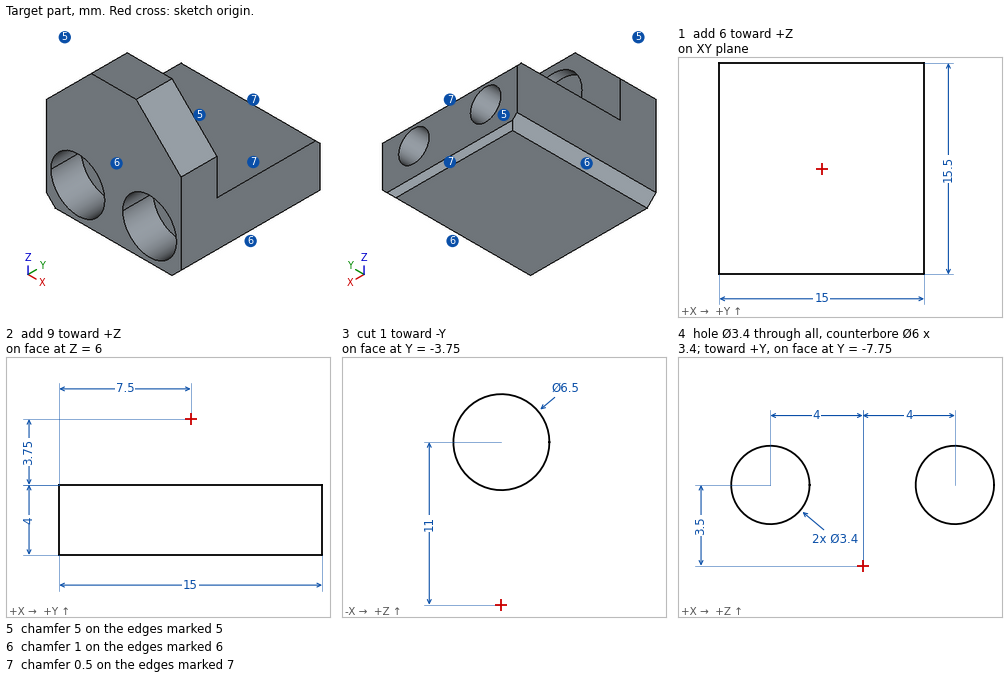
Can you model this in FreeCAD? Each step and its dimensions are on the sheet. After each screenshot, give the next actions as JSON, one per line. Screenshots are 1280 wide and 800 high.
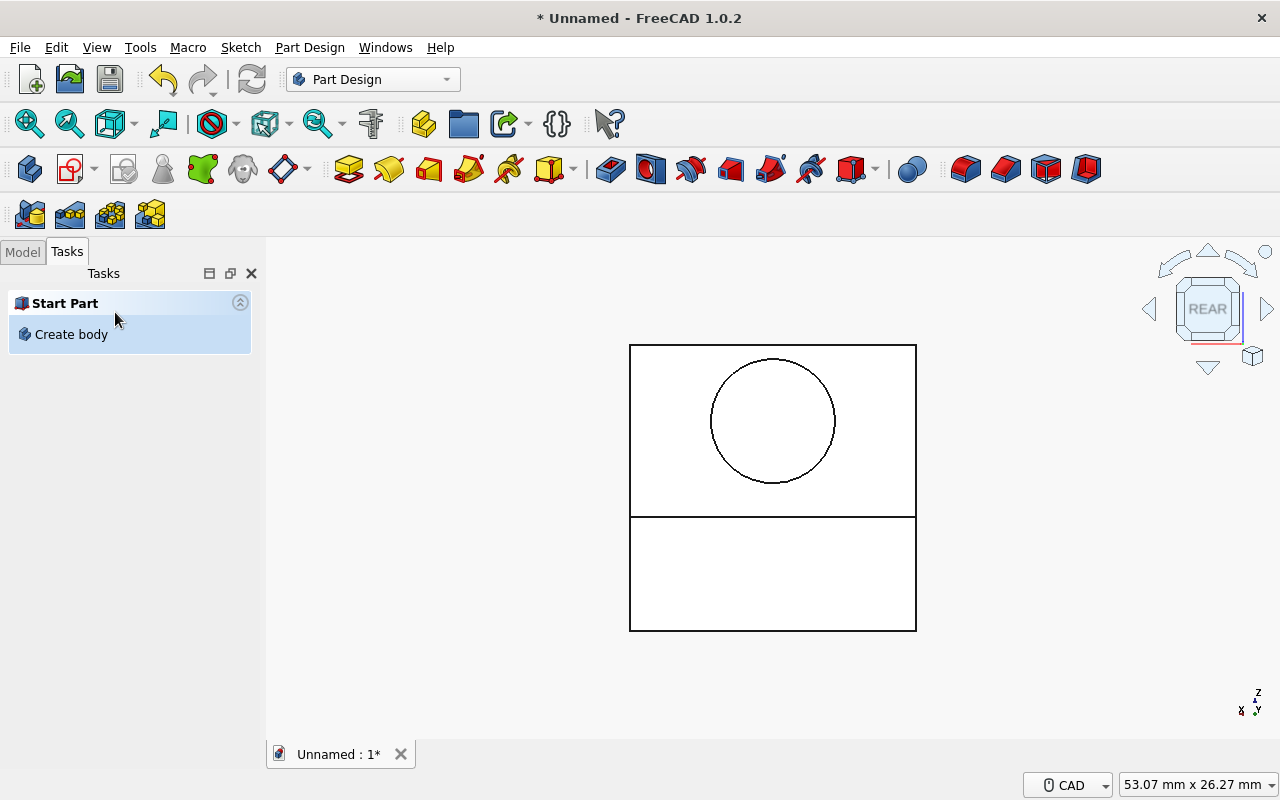
{"action": "key", "text": "0"}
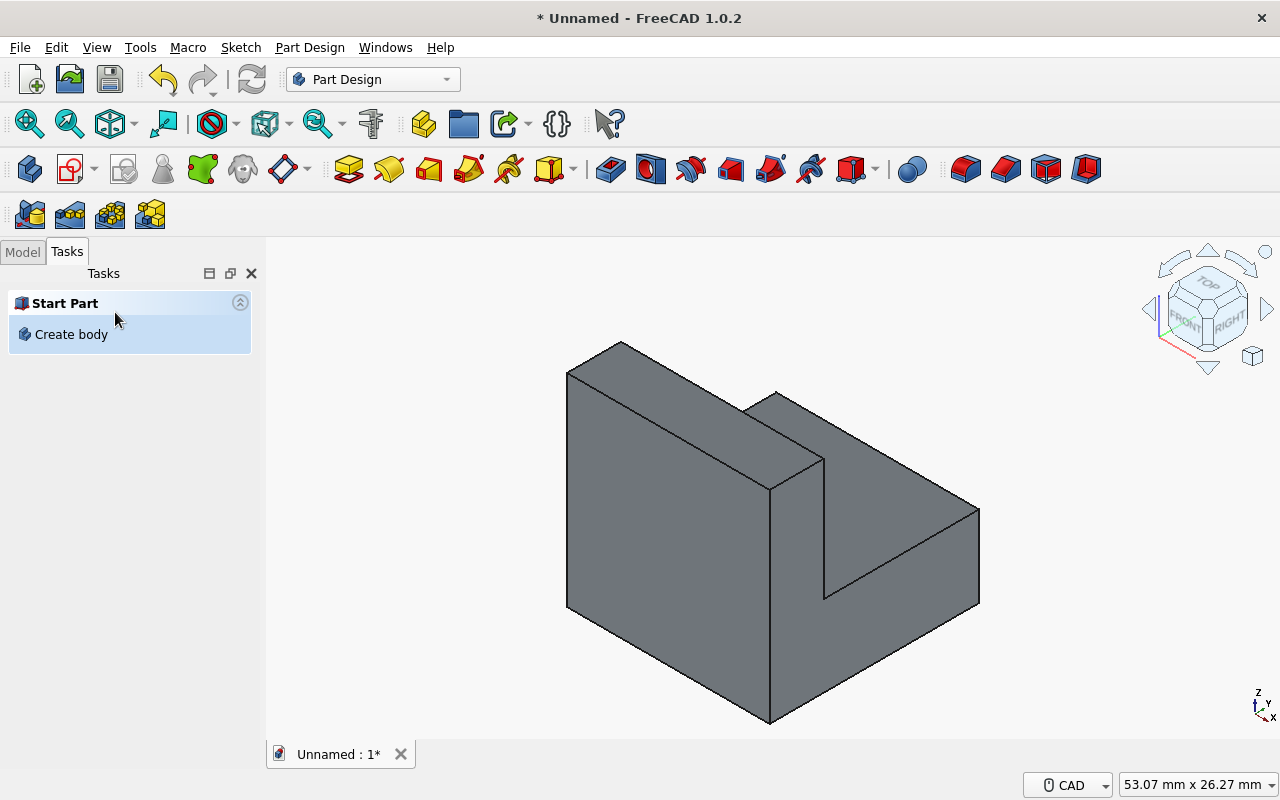
{"action": "left_click", "coordinate": [668, 547]}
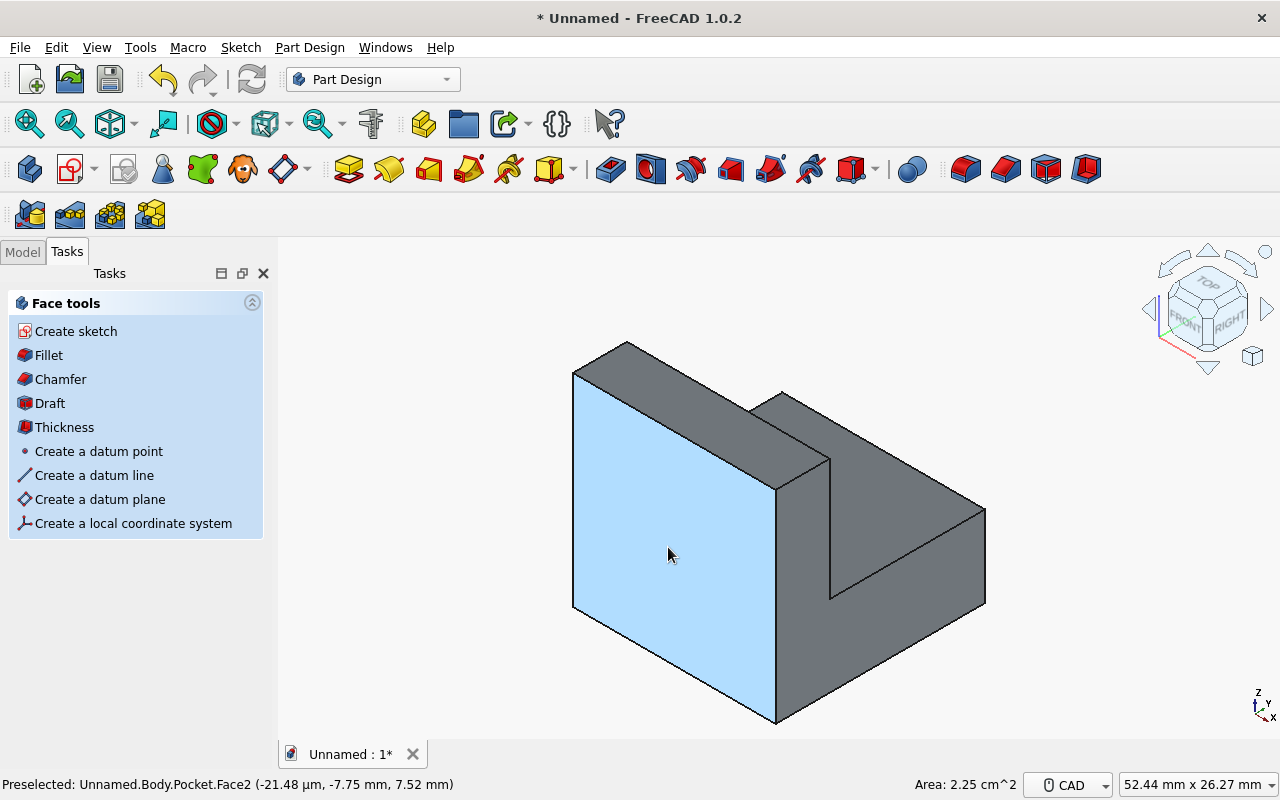
{"action": "left_click", "coordinate": [70, 170]}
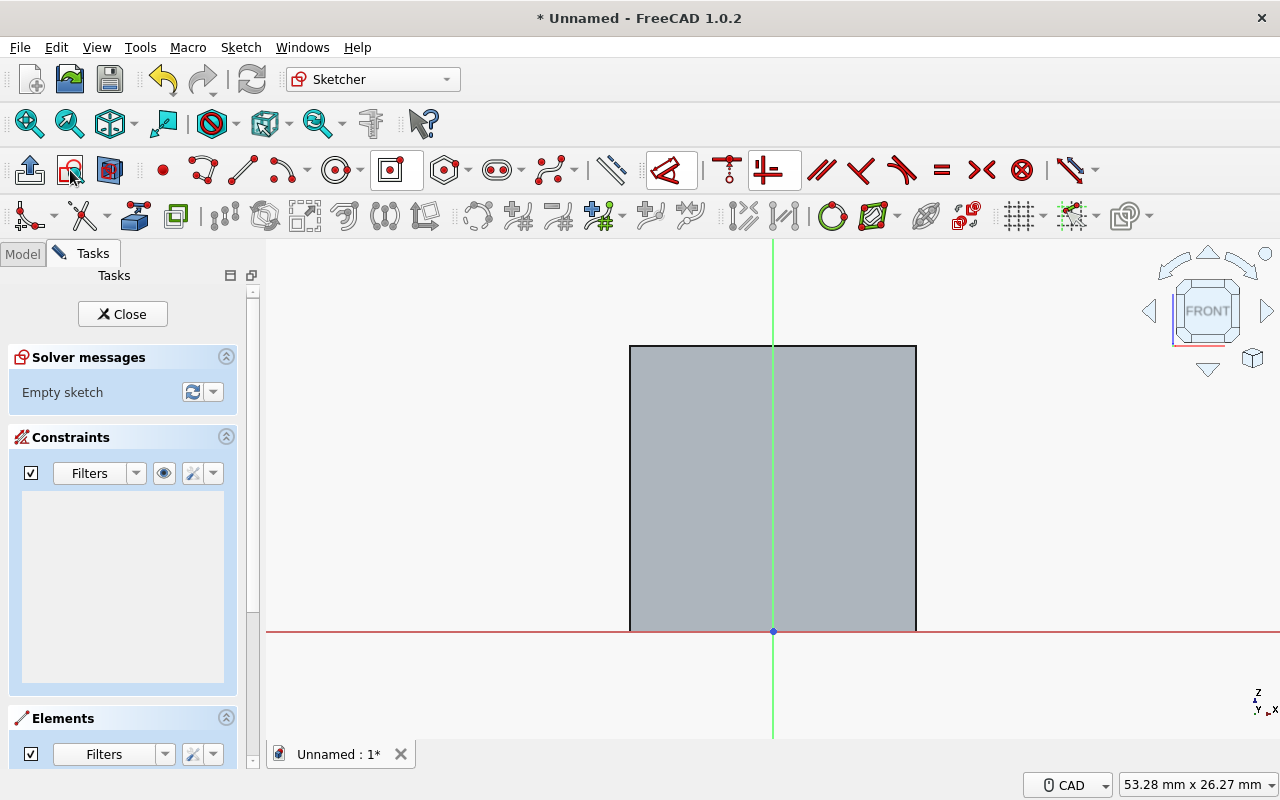
{"action": "scroll", "coordinate": [813, 637], "scroll_direction": "up", "scroll_amount": 5}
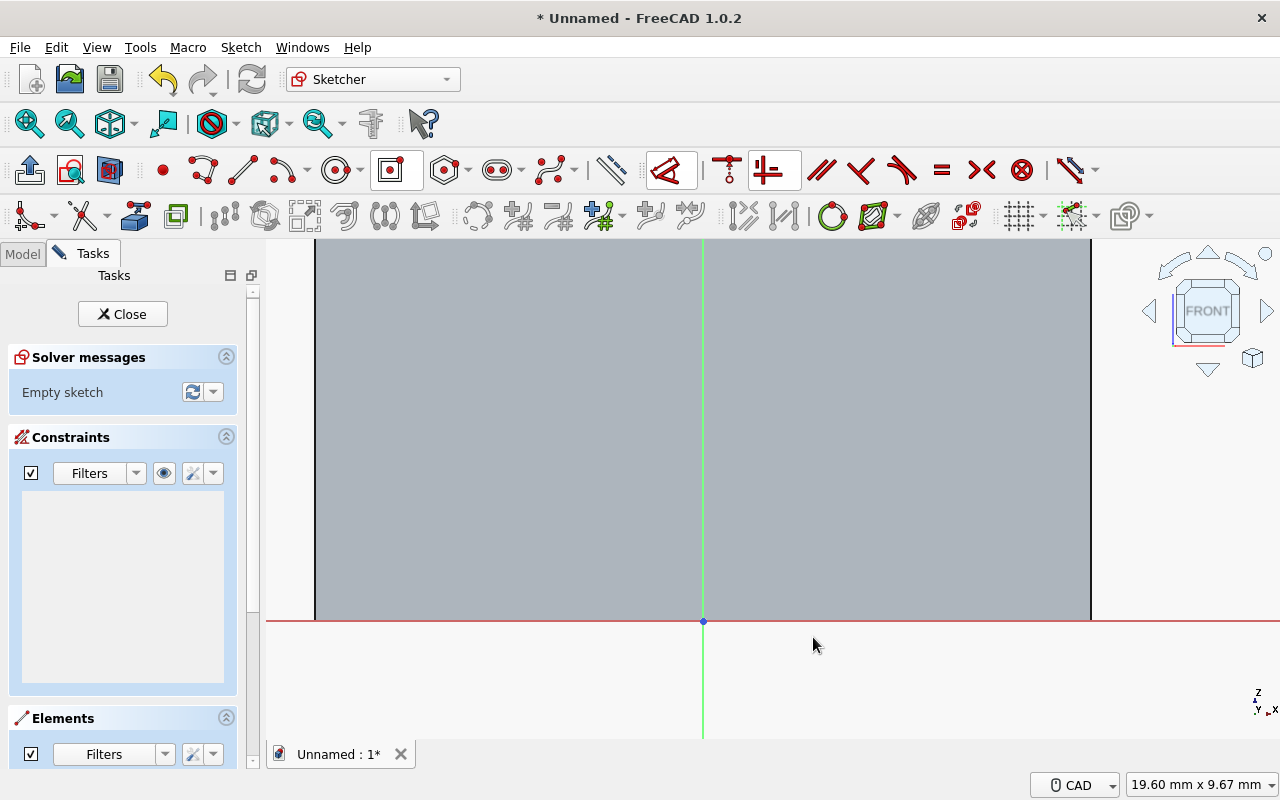
{"action": "left_click", "coordinate": [336, 170]}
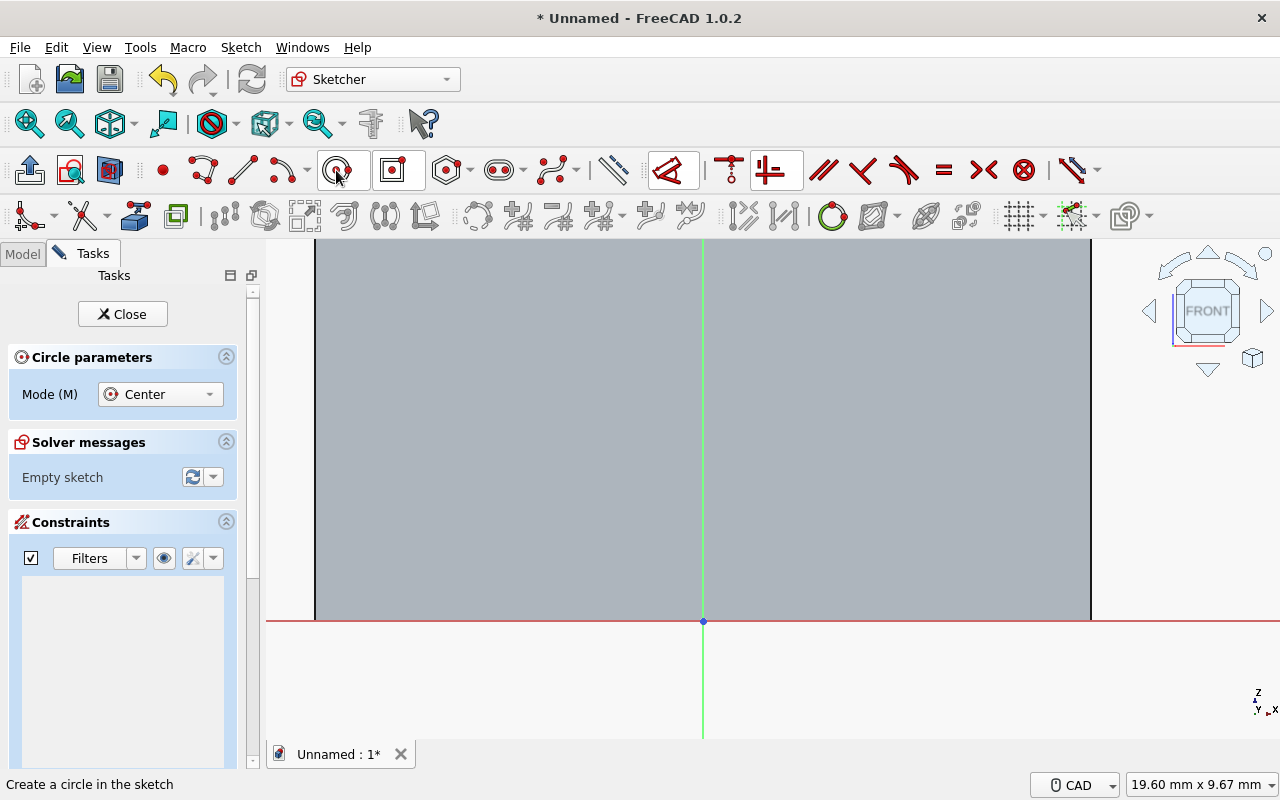
{"action": "left_click", "coordinate": [496, 440]}
{"action": "left_click", "coordinate": [559, 378]}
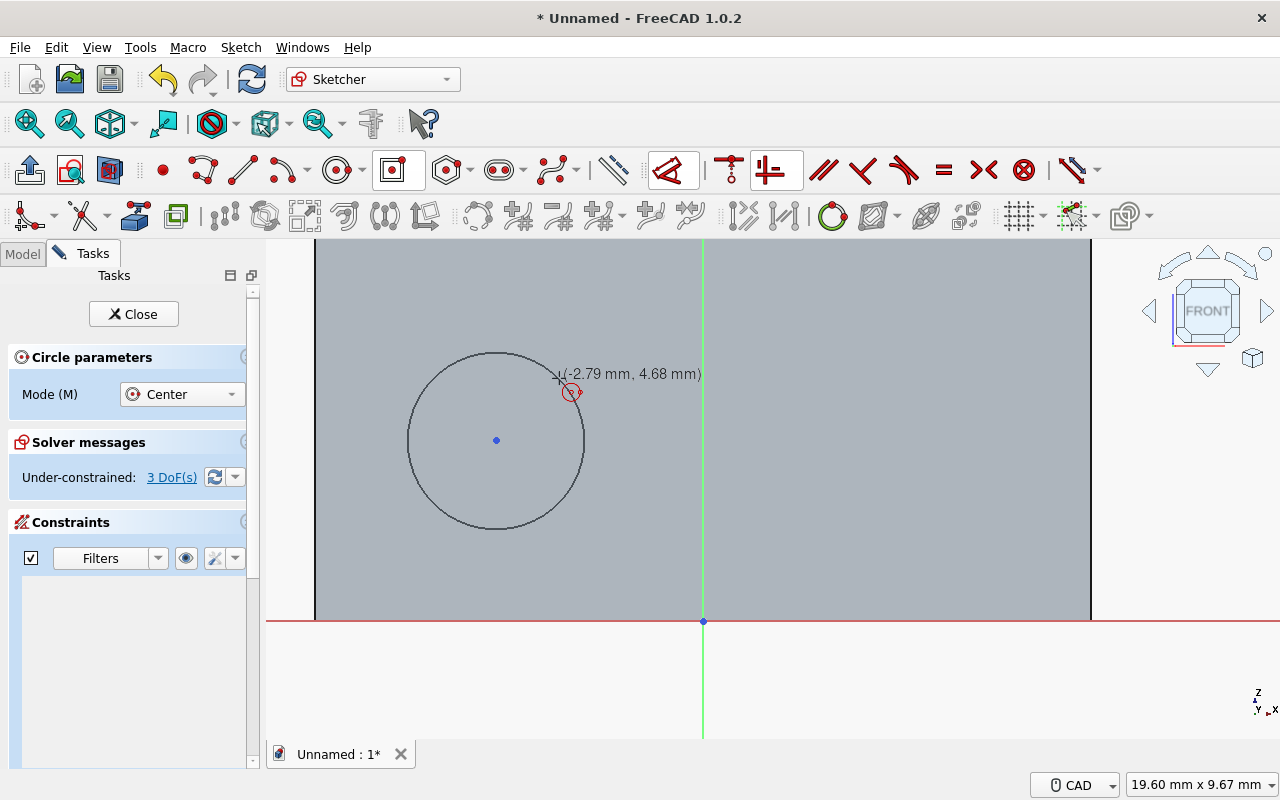
{"action": "left_click", "coordinate": [910, 440]}
{"action": "left_click", "coordinate": [972, 378]}
{"action": "key", "text": "Escape"}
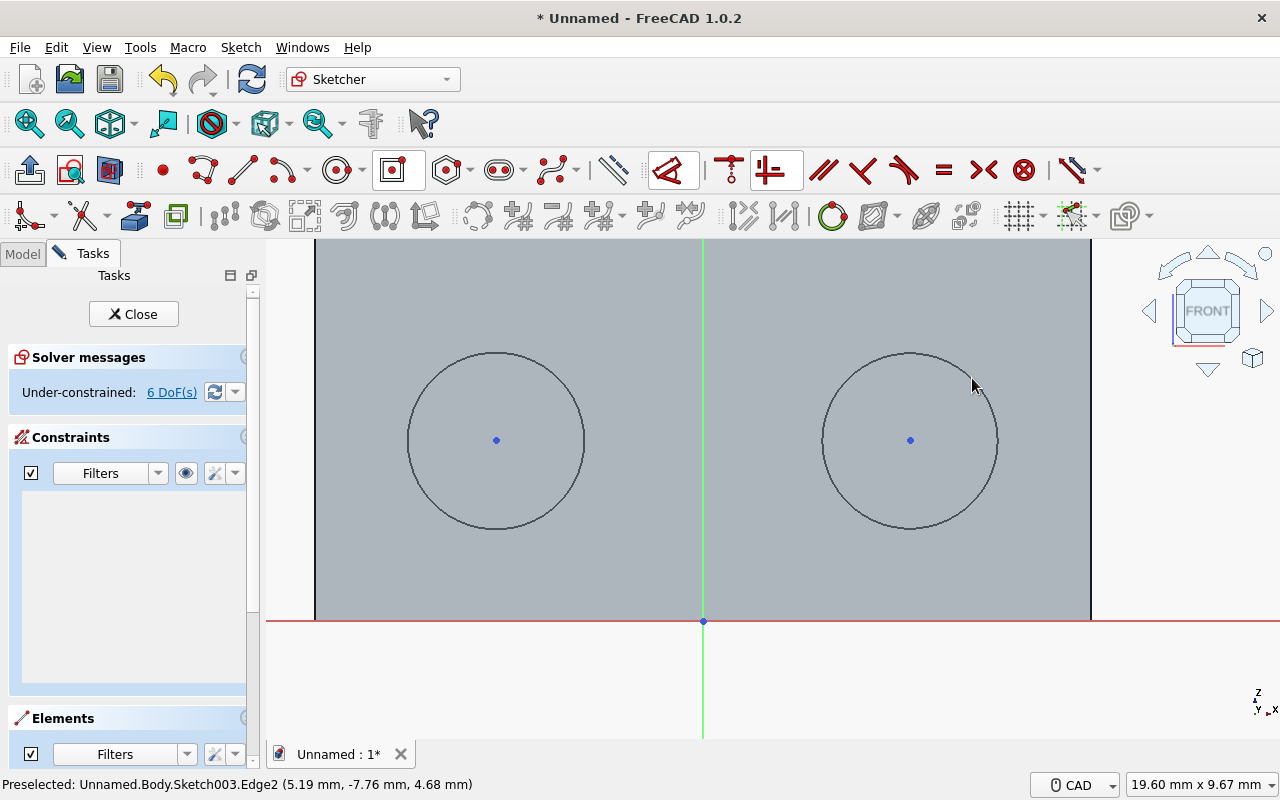
{"action": "left_click", "coordinate": [558, 378]}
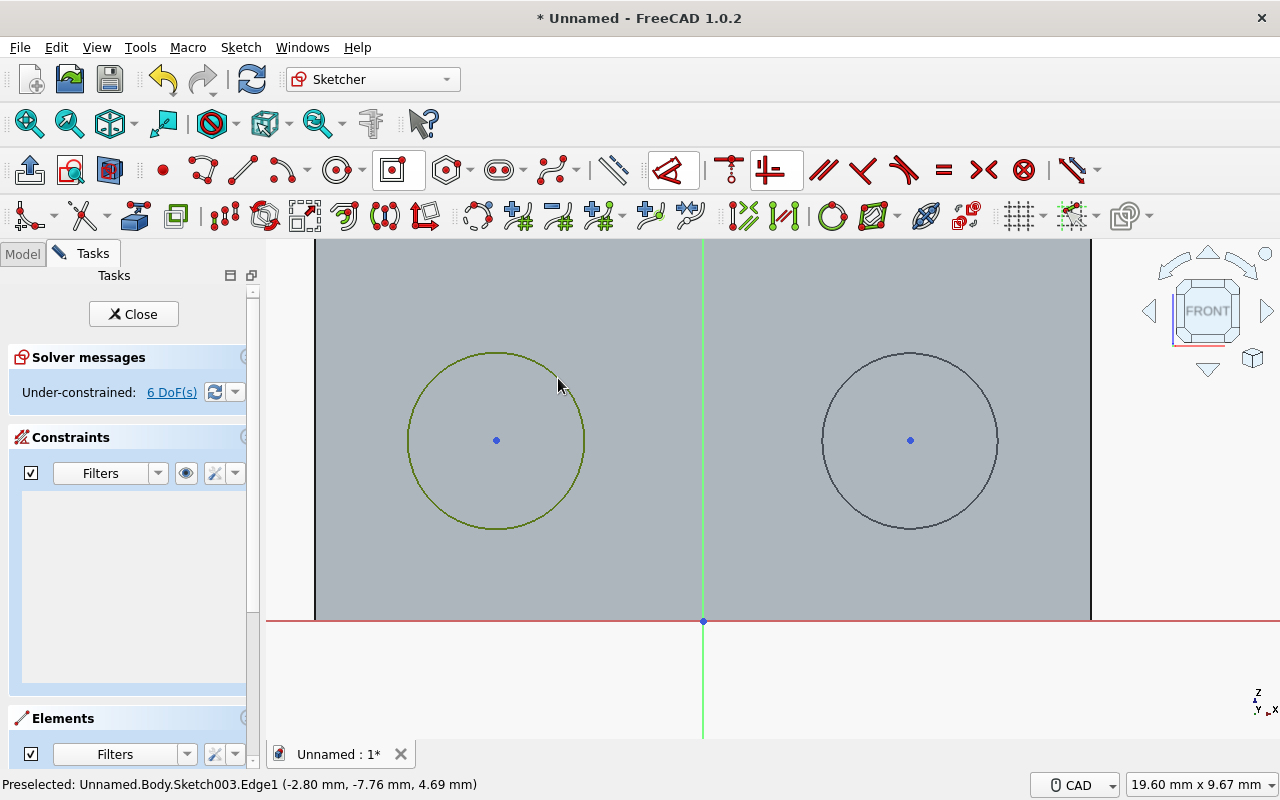
{"action": "left_click", "coordinate": [972, 379]}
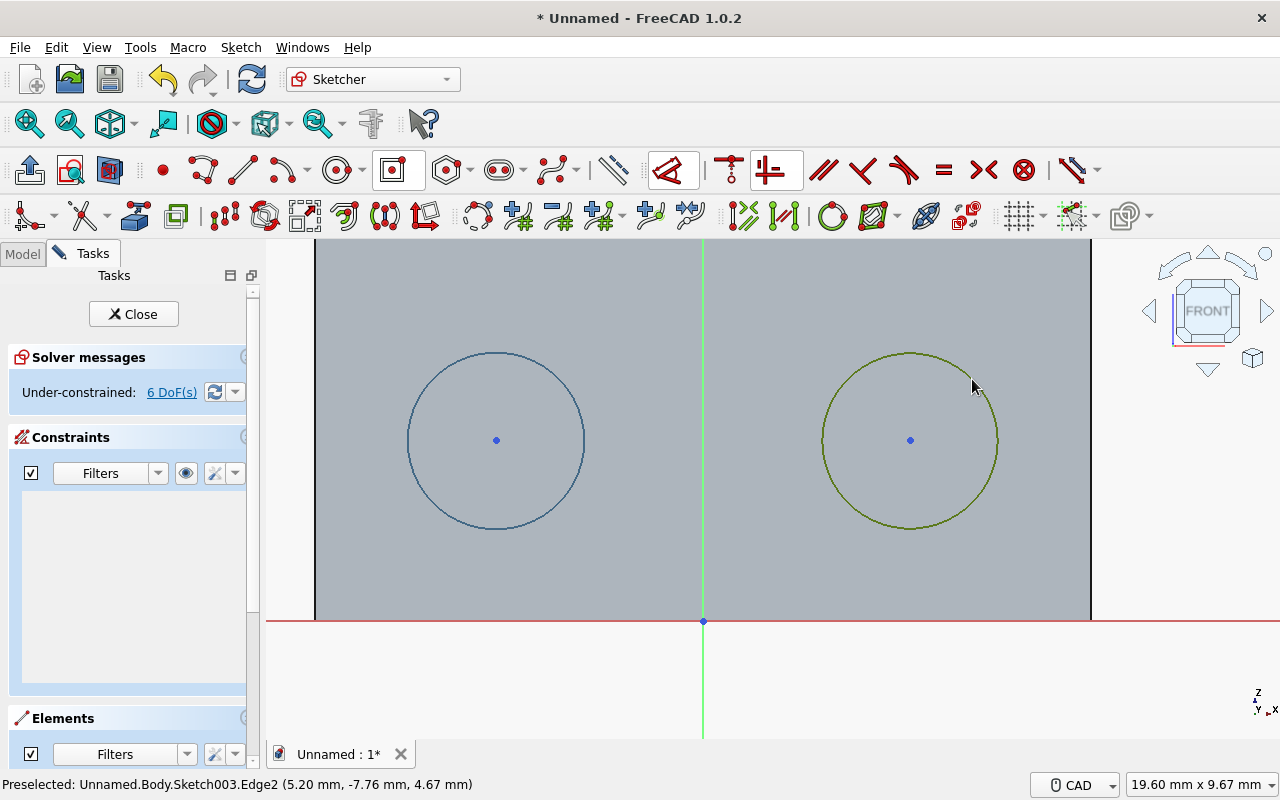
{"action": "key", "text": "e"}